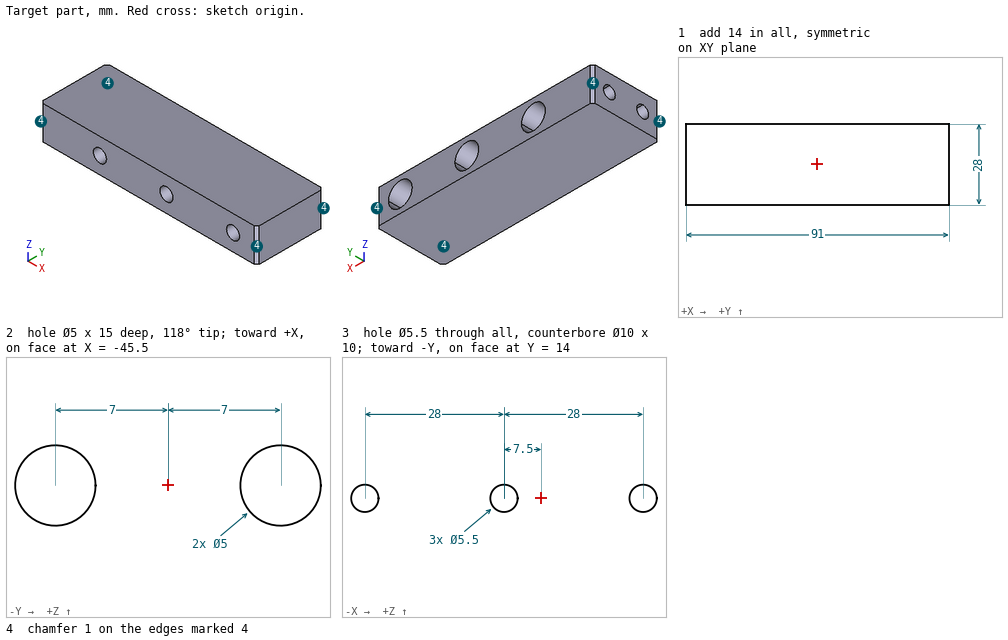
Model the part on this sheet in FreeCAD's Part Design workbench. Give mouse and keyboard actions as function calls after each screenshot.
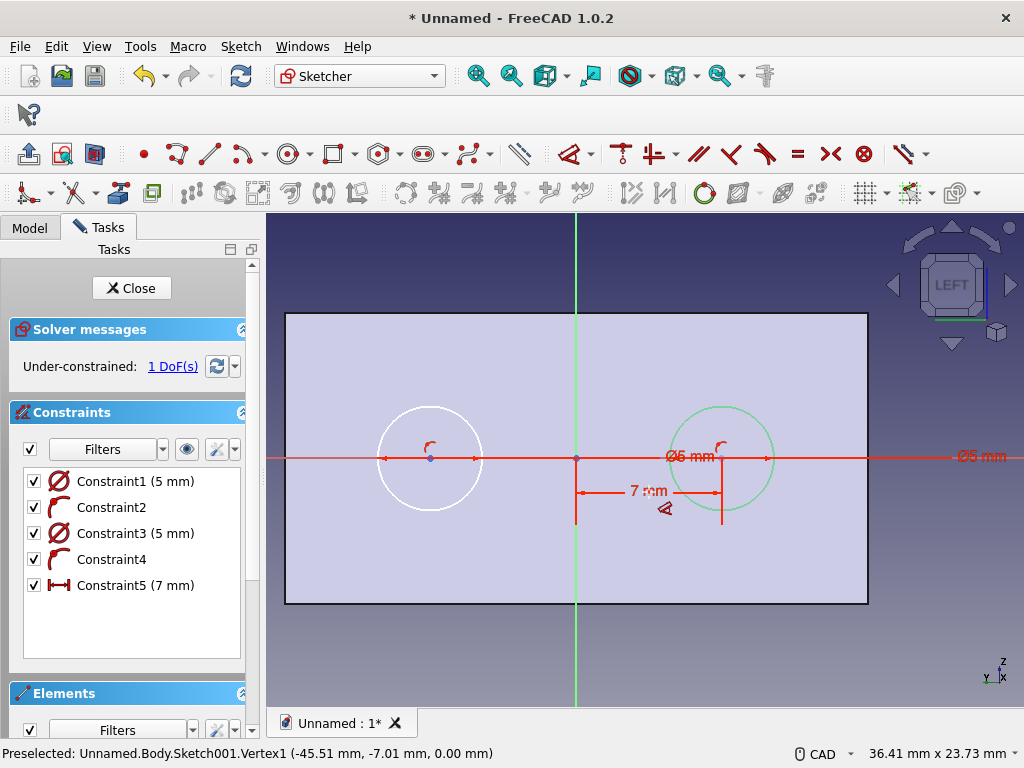
click(430, 458)
click(503, 492)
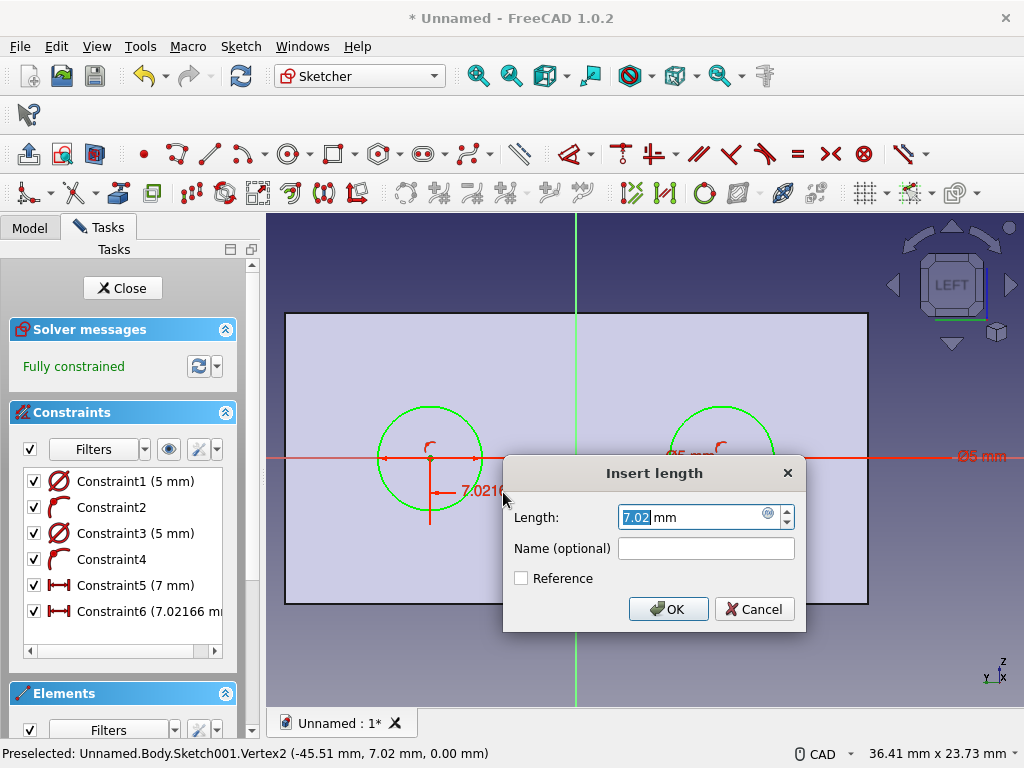
text(7)
key(Return)
key(Escape)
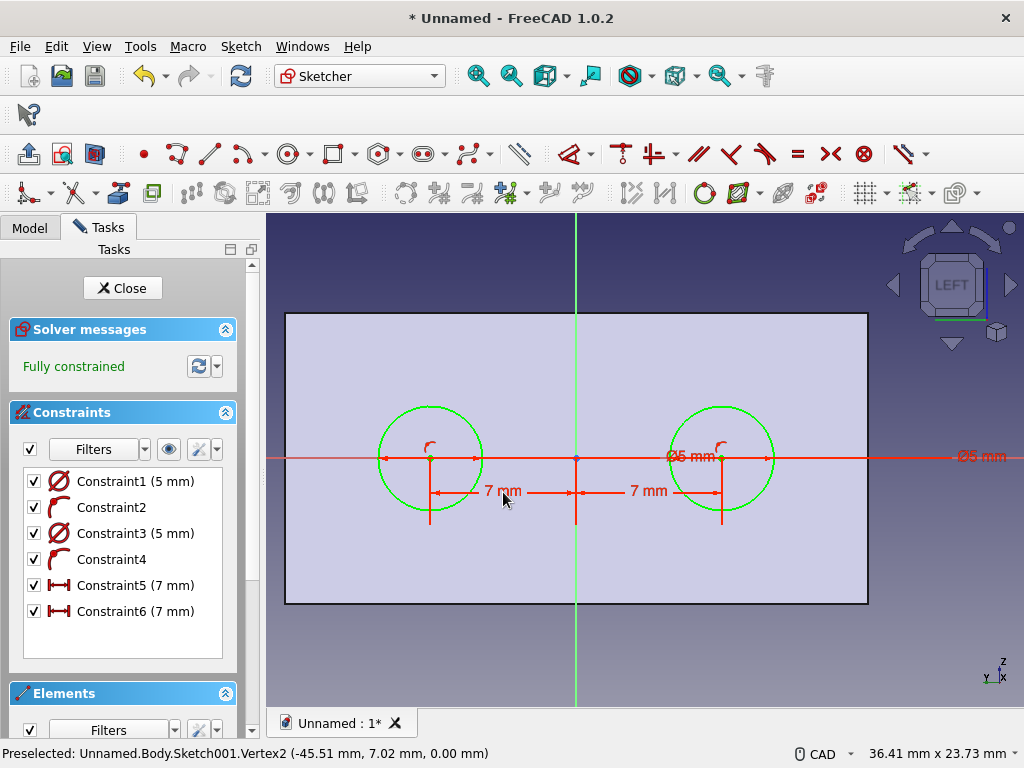
click(123, 288)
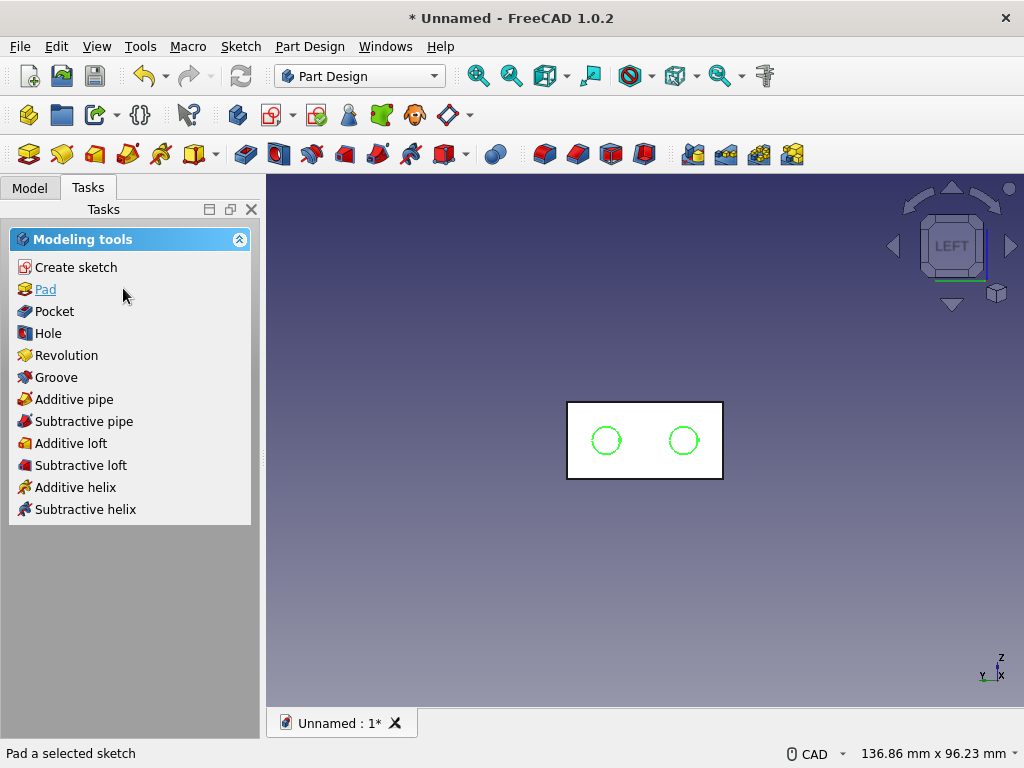
click(279, 154)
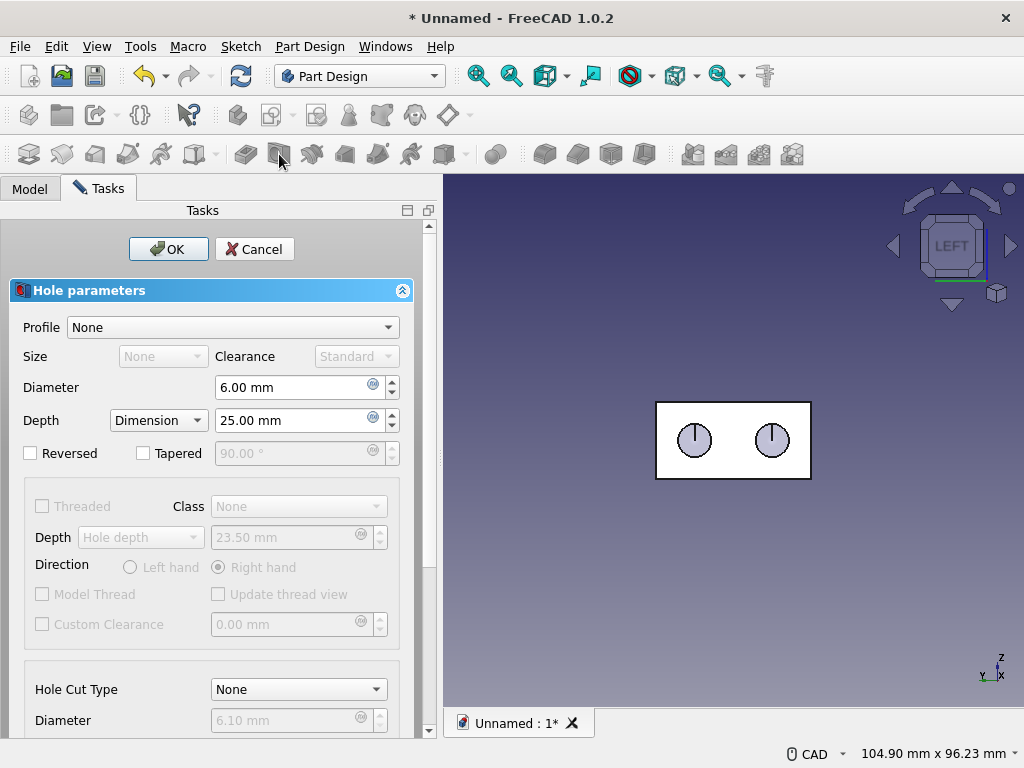
triple_click(300, 388)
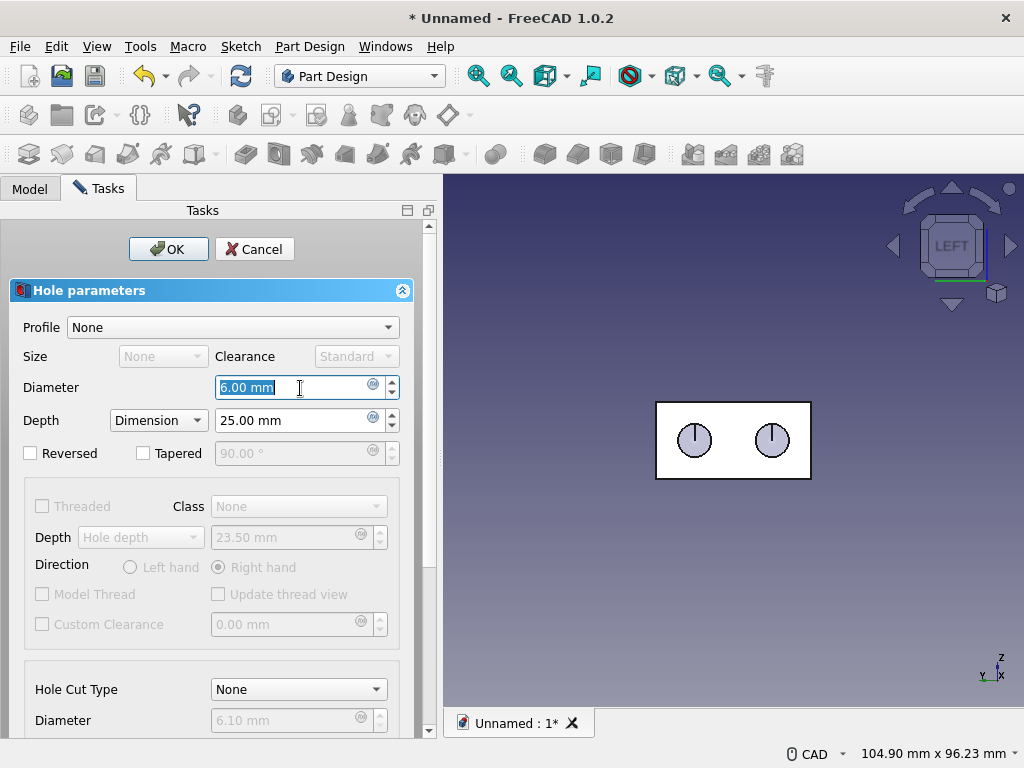
text(5)
key(Tab)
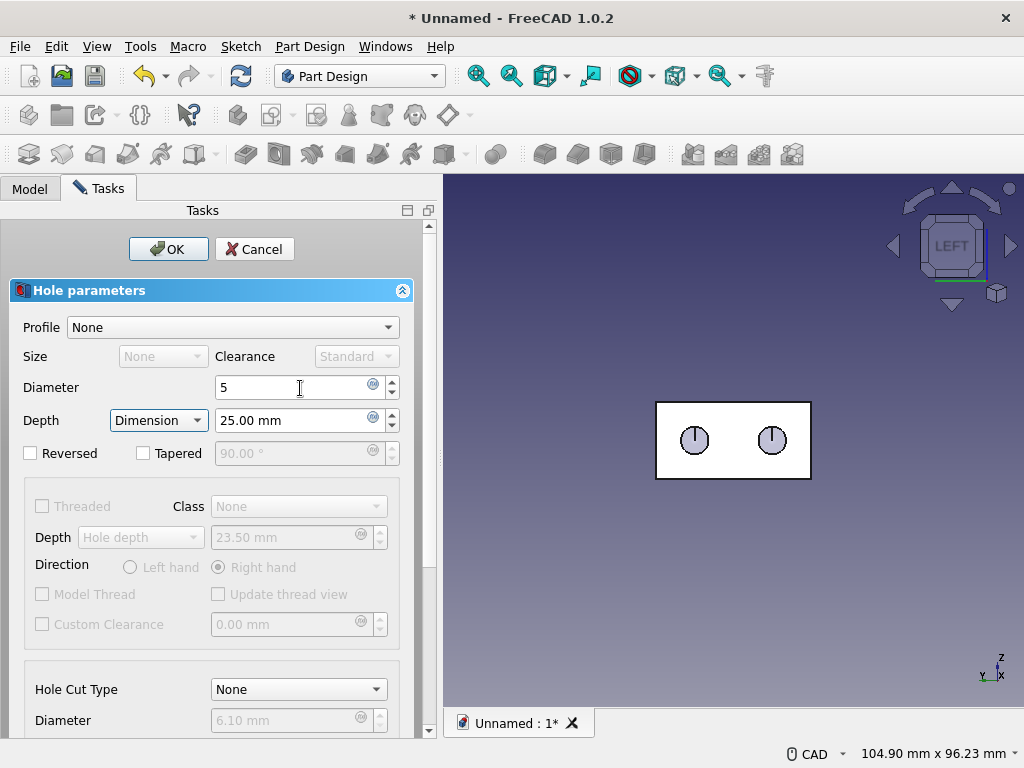
triple_click(300, 420)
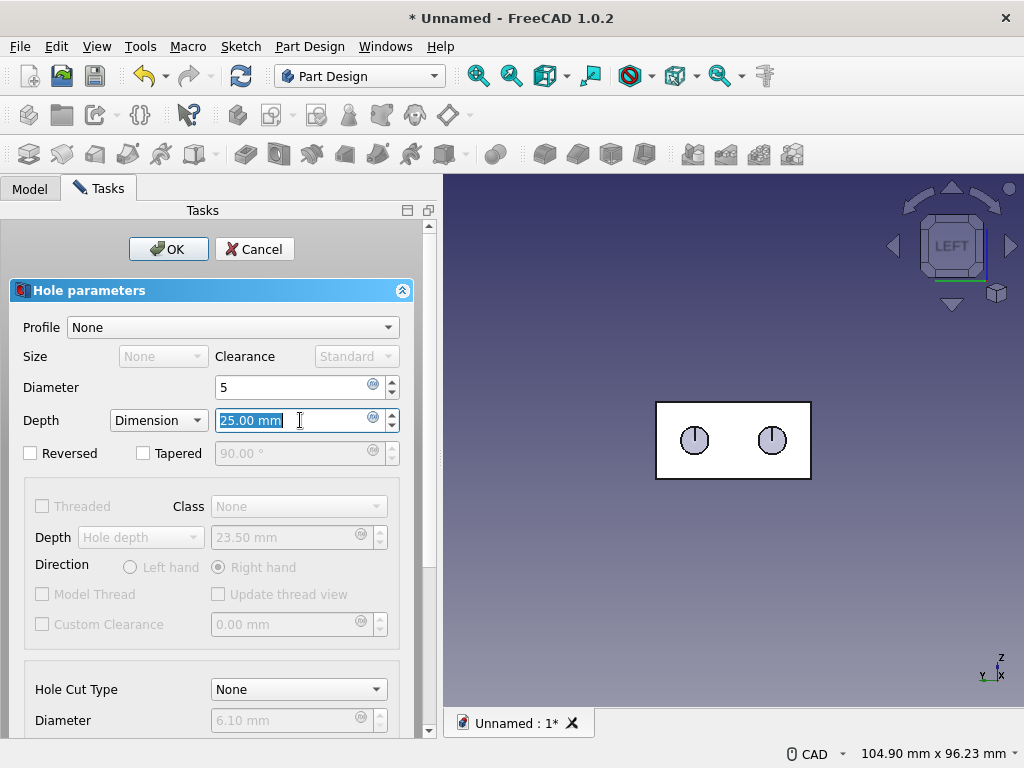
text(15)
key(Tab)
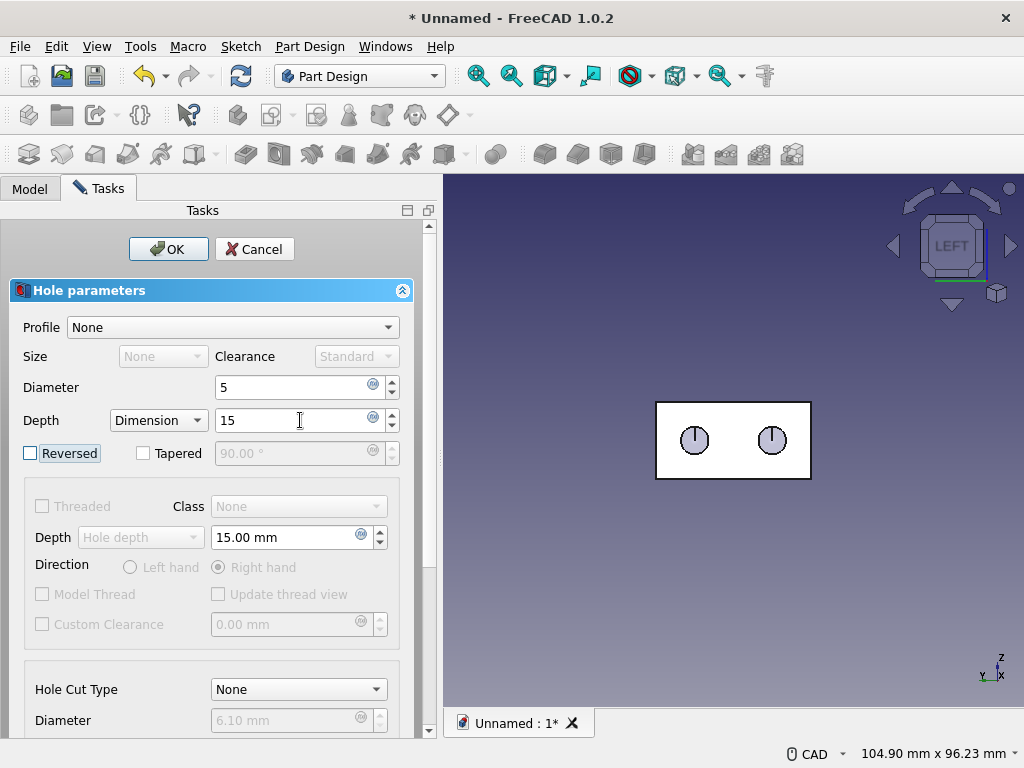
click(169, 249)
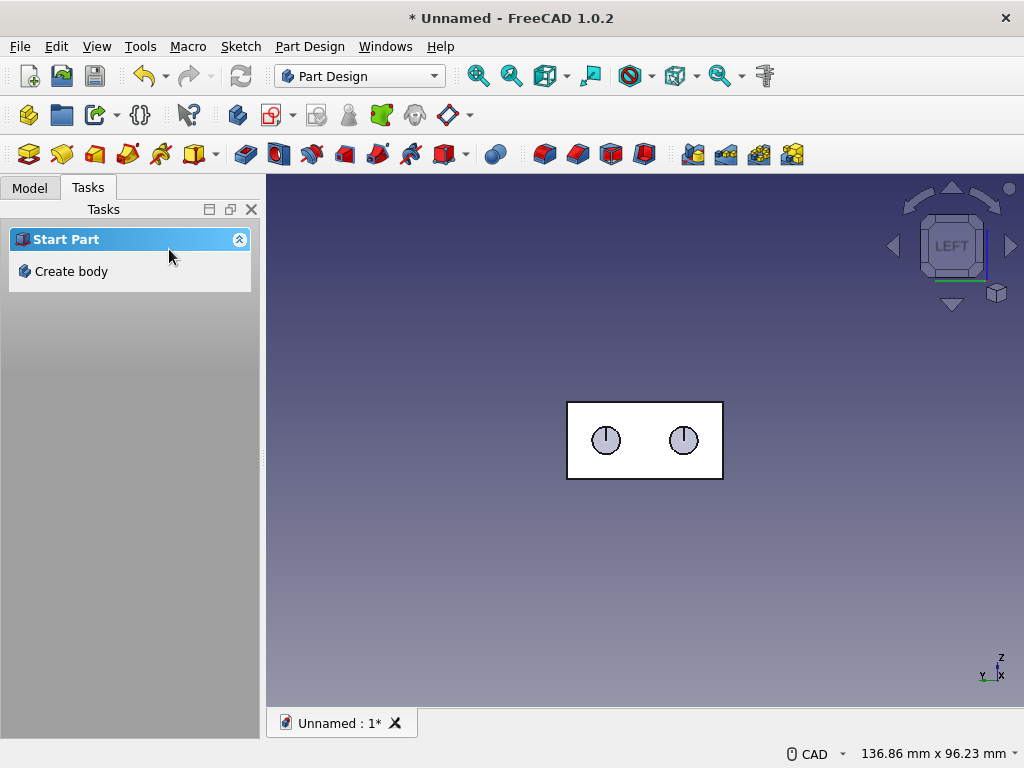
key(v)
key(f)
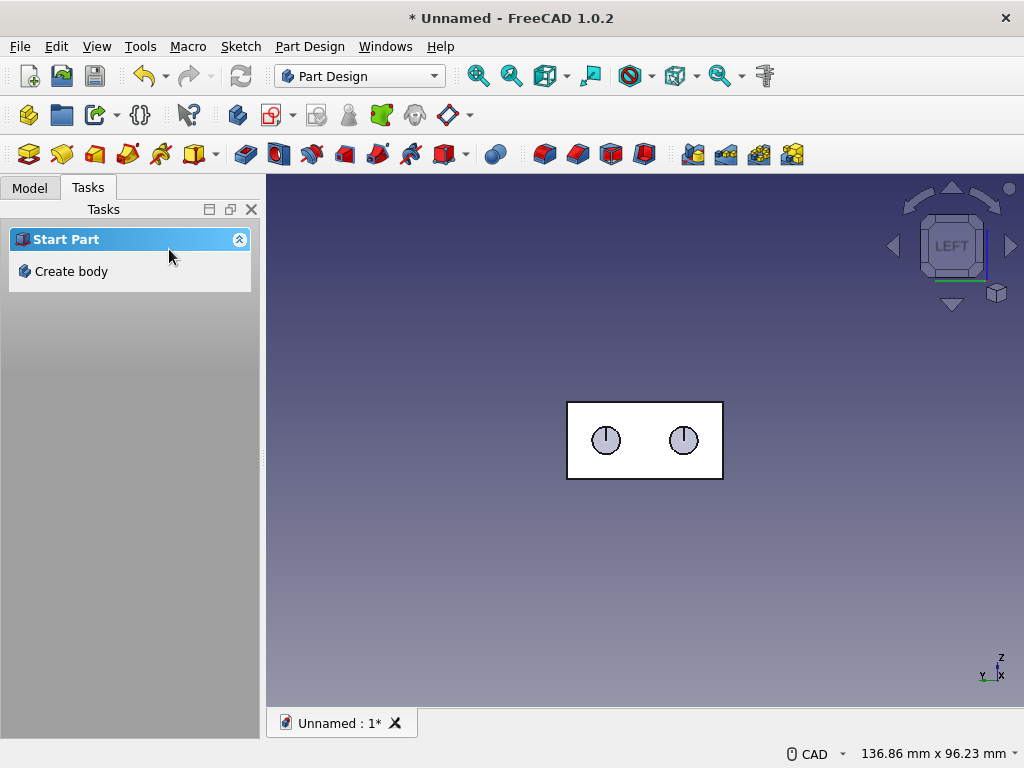
key(4)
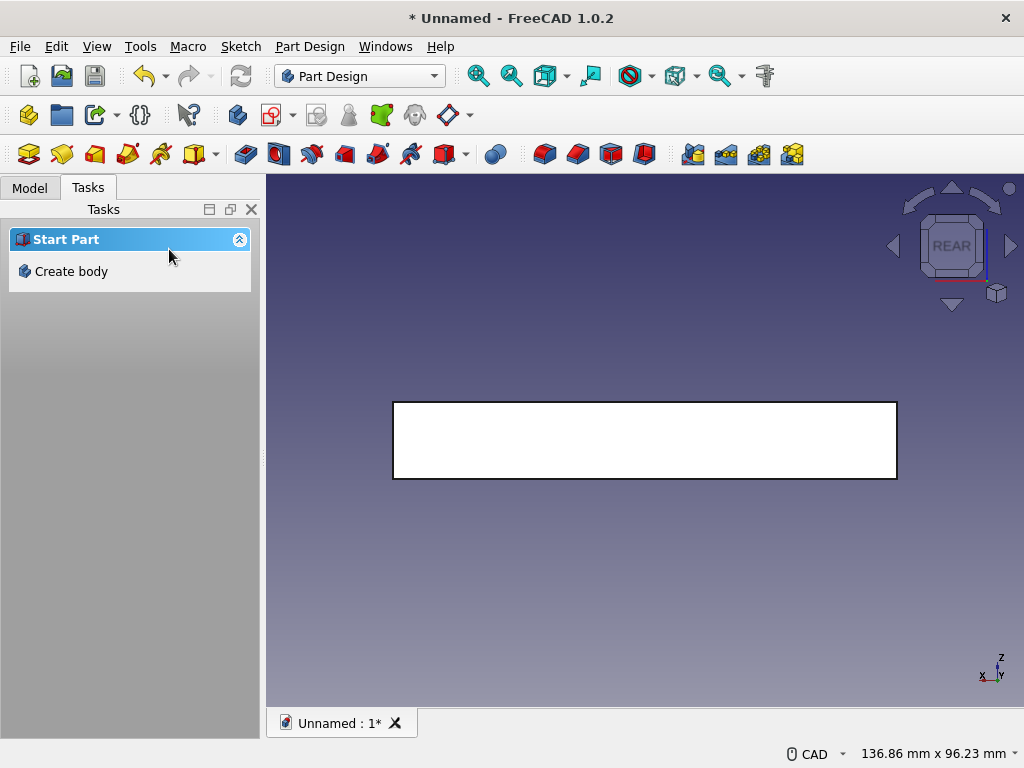
click(501, 440)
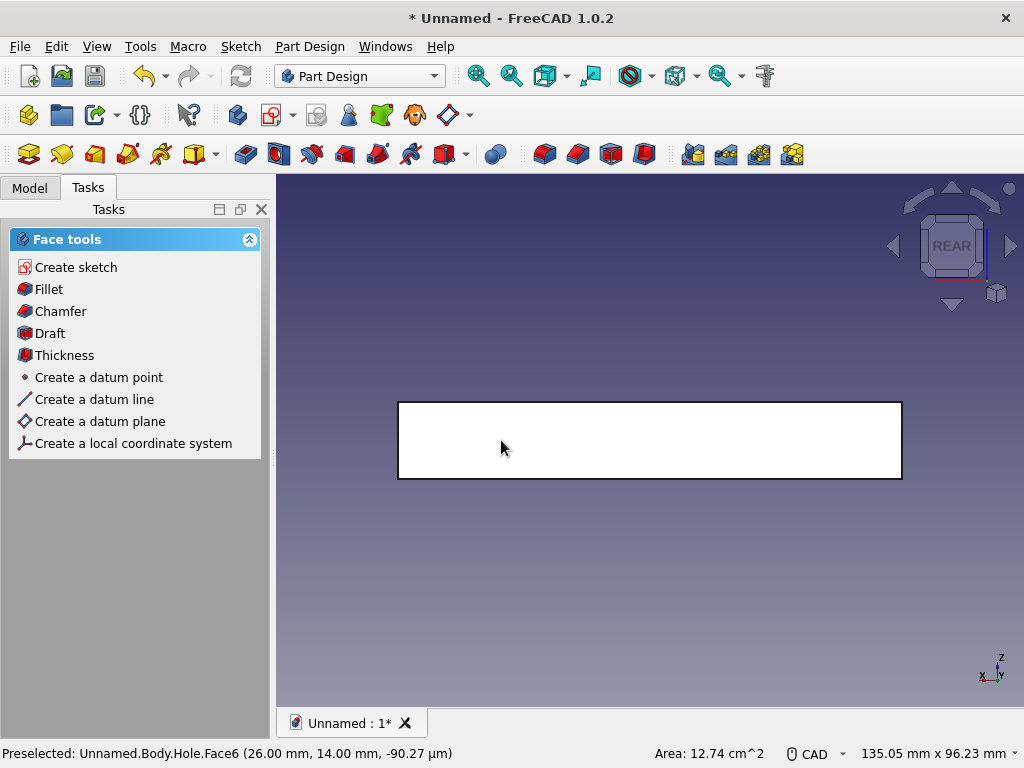
click(270, 116)